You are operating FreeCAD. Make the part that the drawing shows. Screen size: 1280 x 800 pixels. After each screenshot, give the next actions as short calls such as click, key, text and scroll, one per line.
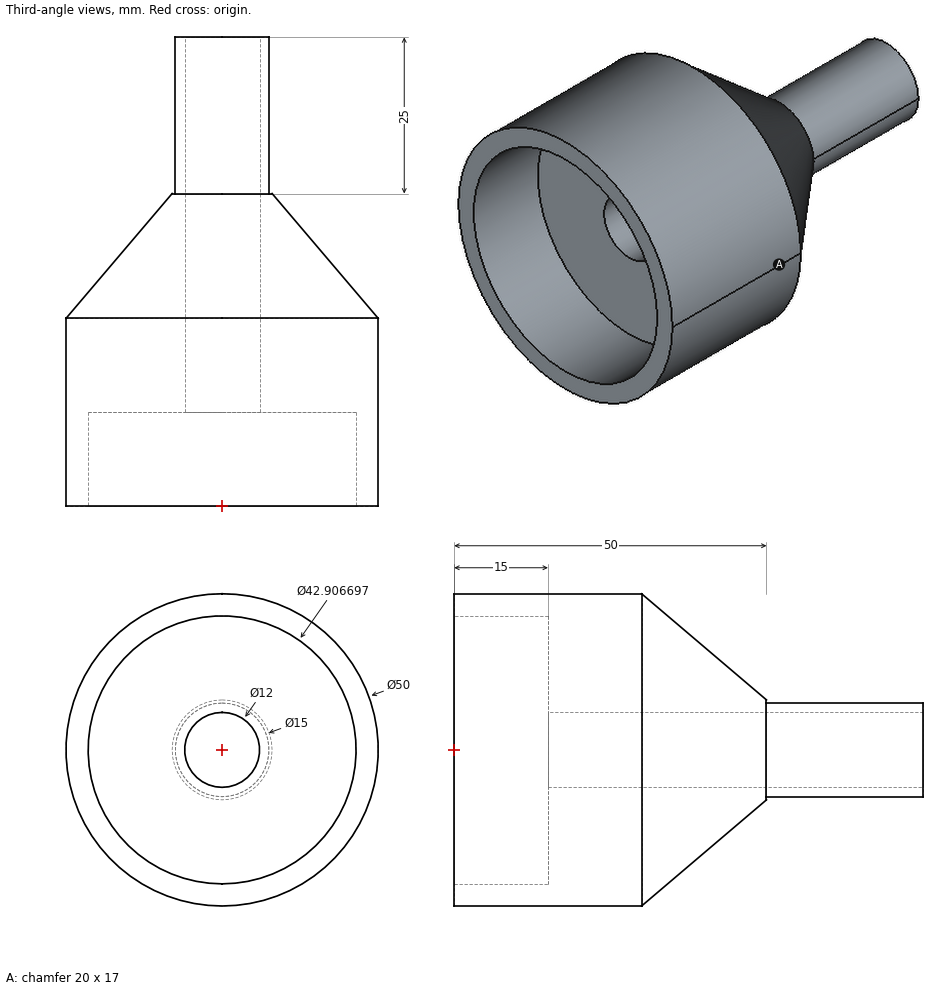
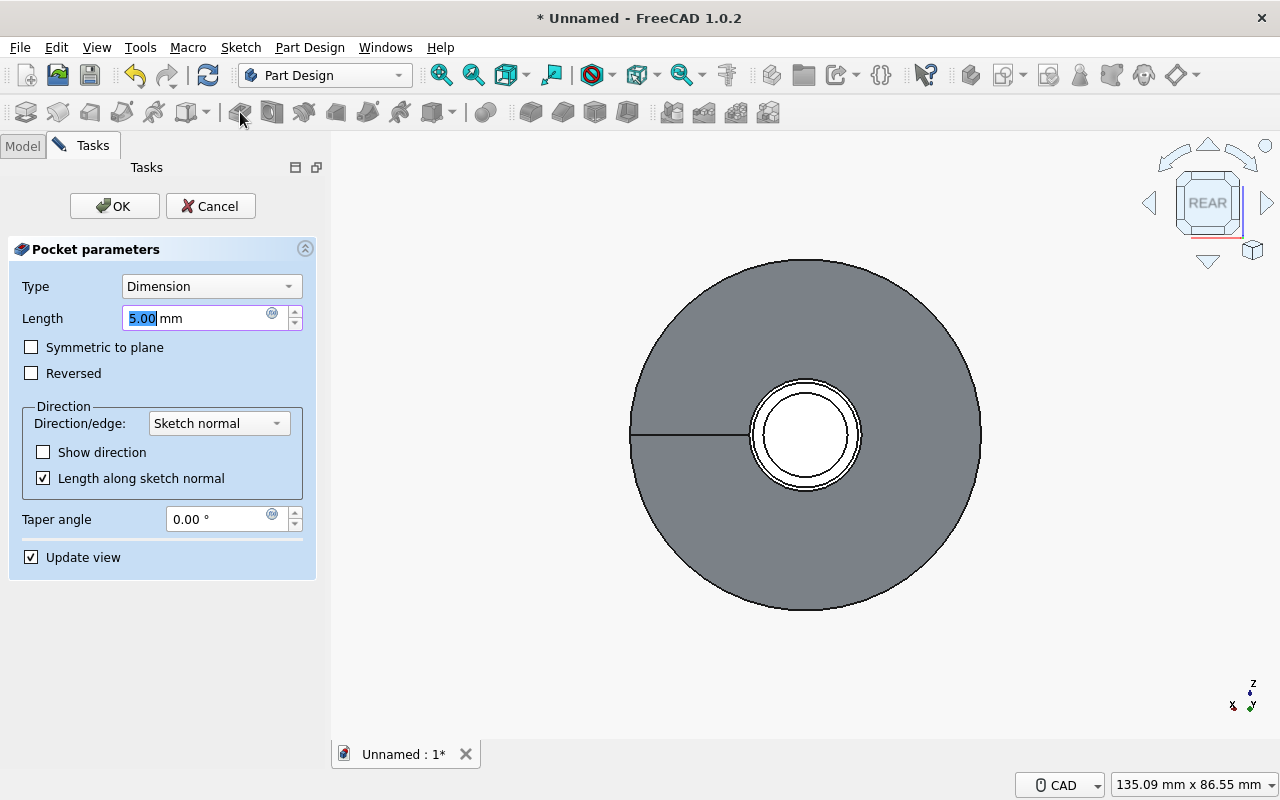
click(212, 286)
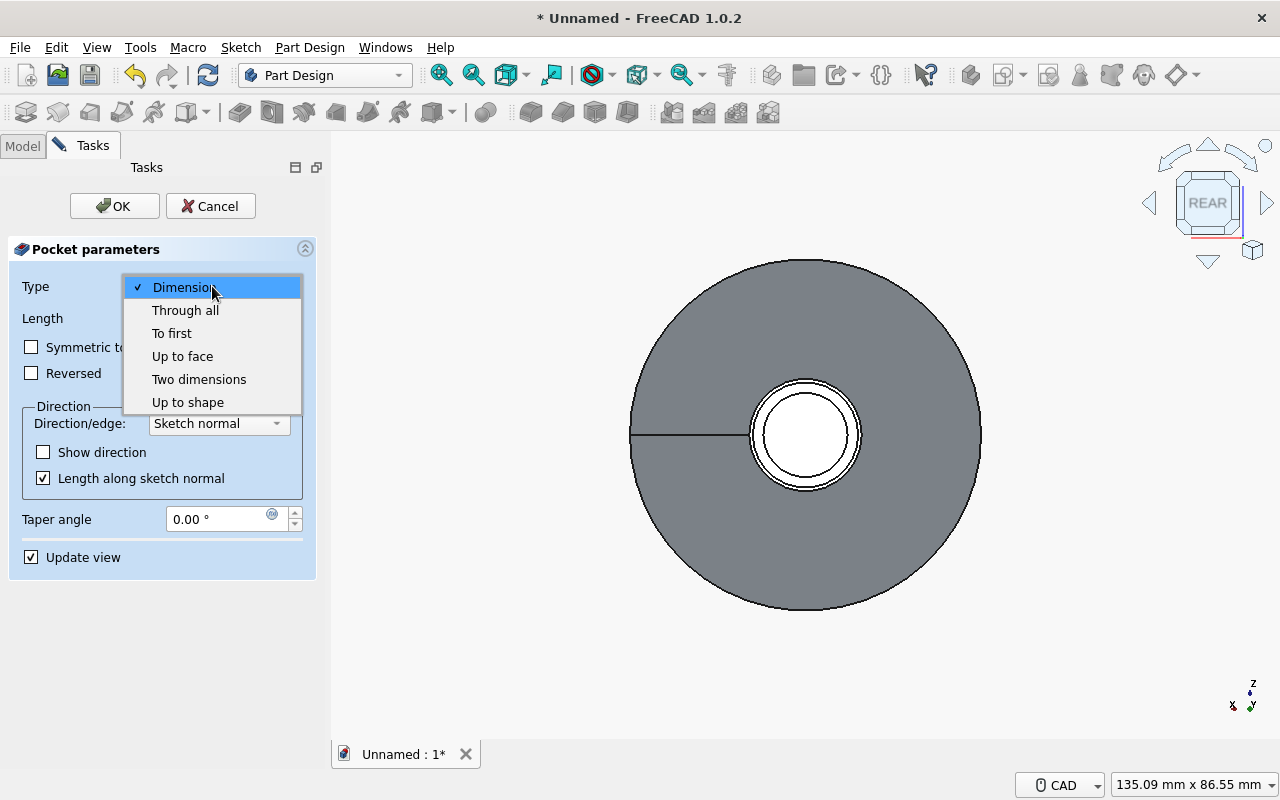
click(212, 310)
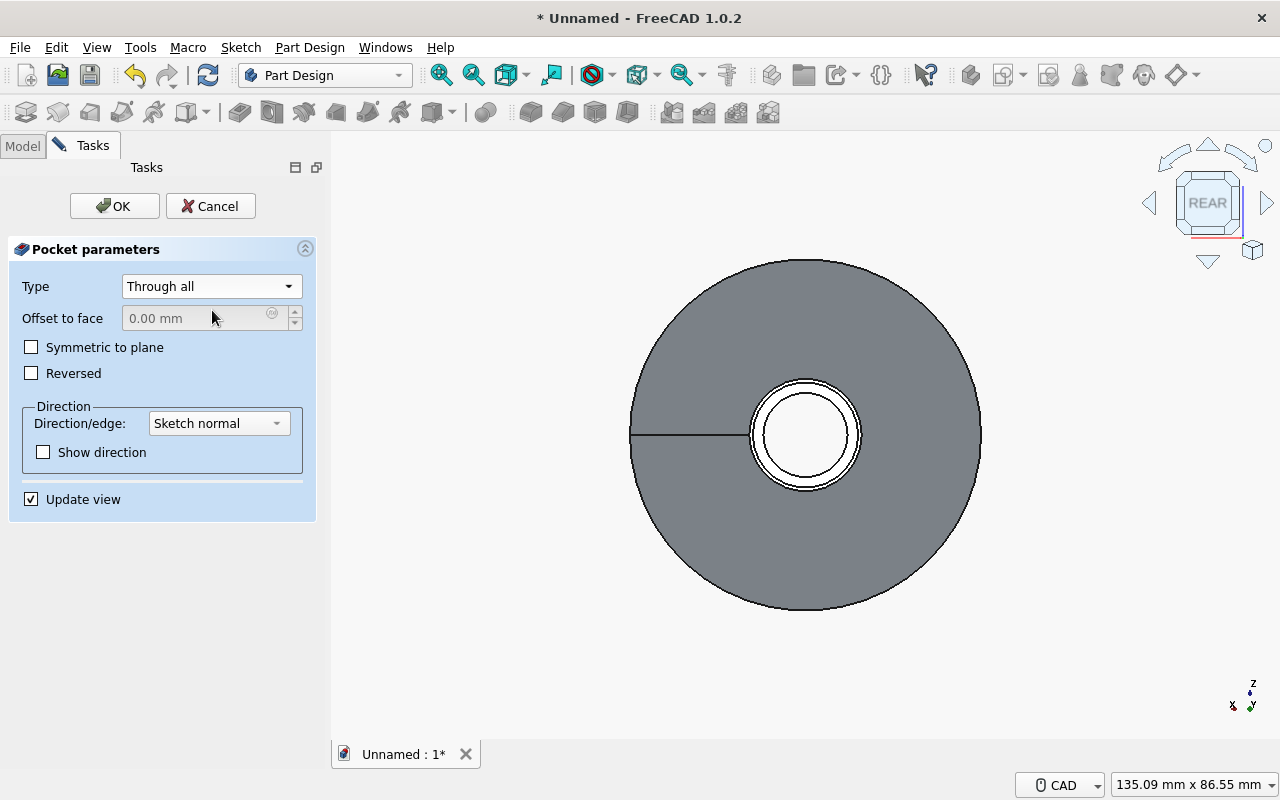
click(115, 206)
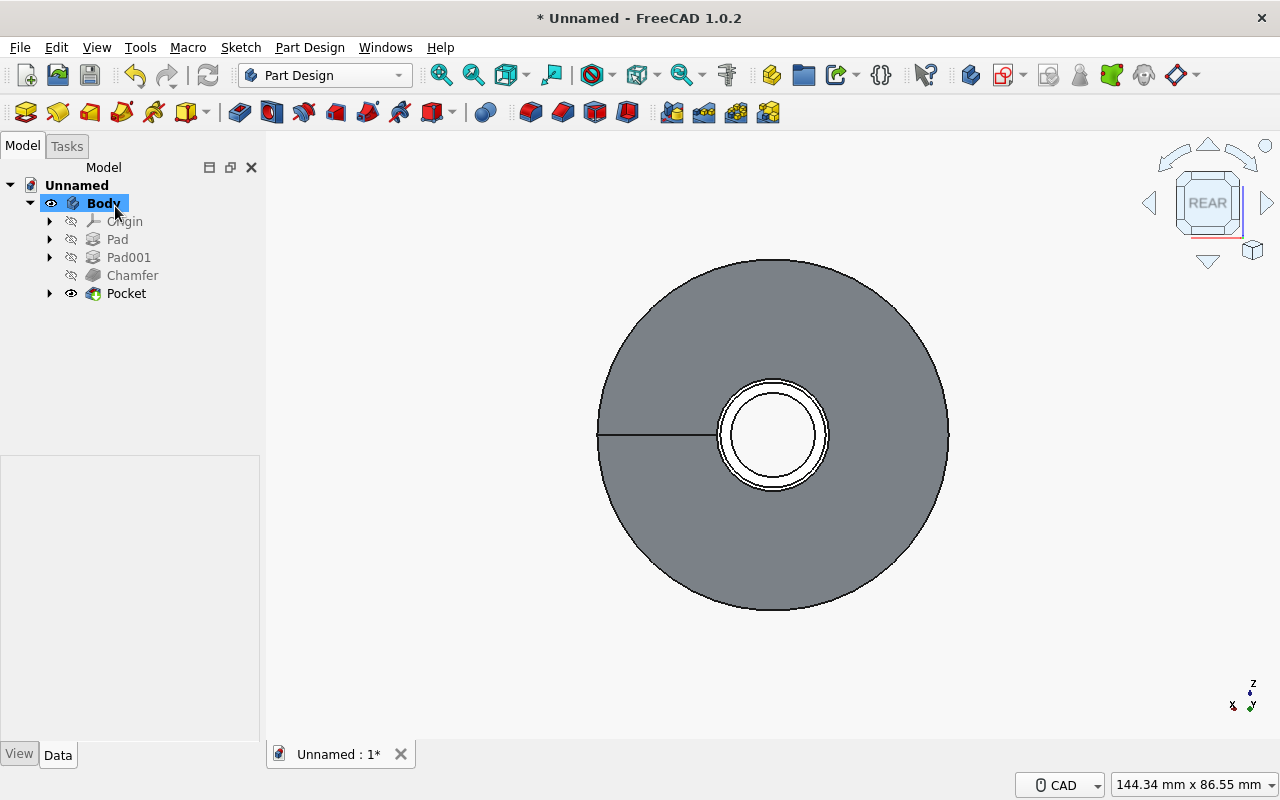
click(1004, 76)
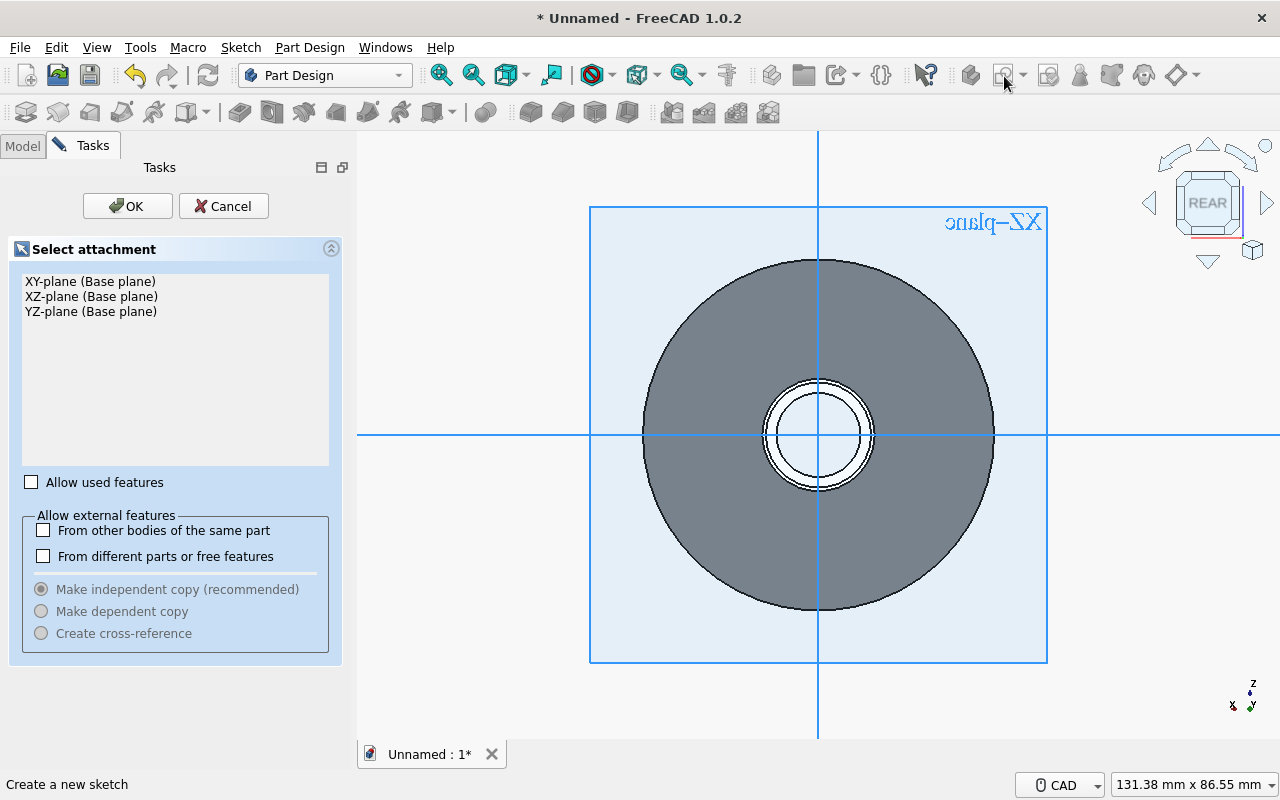
click(82, 296)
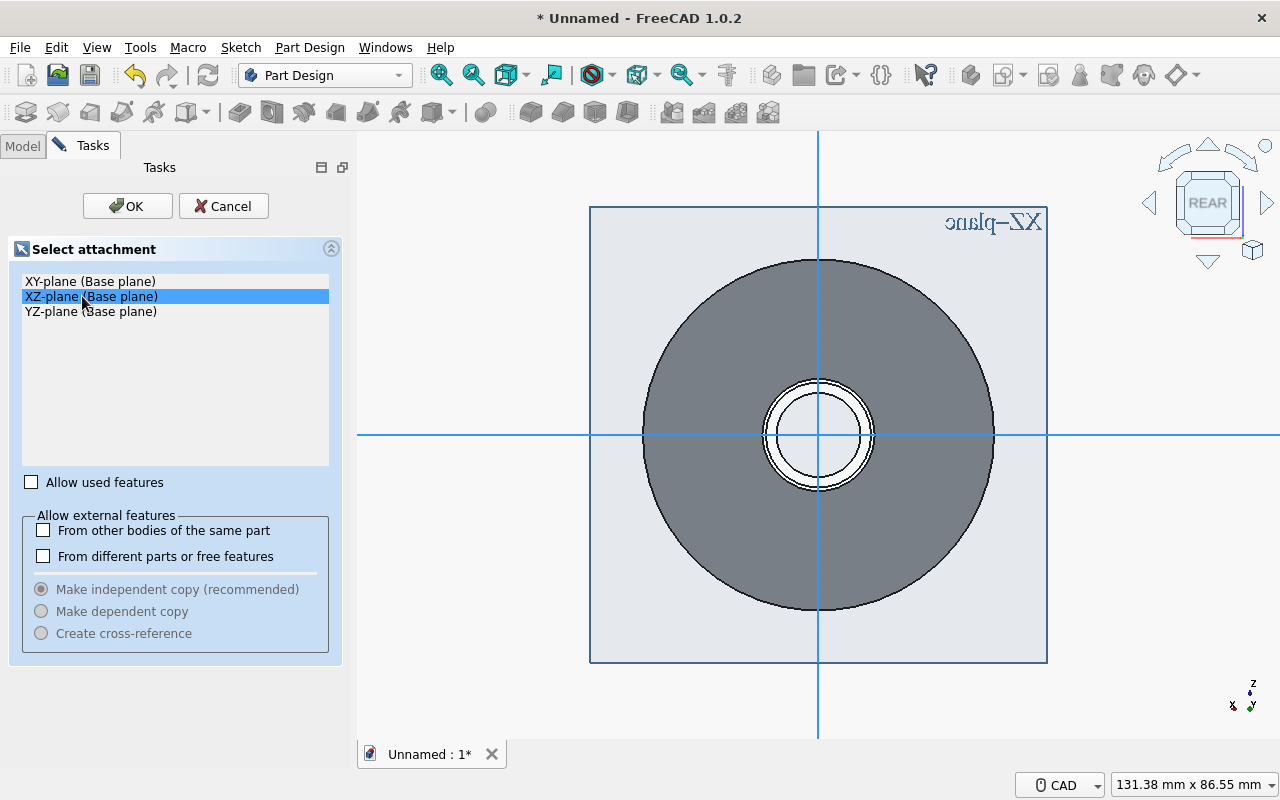
click(128, 206)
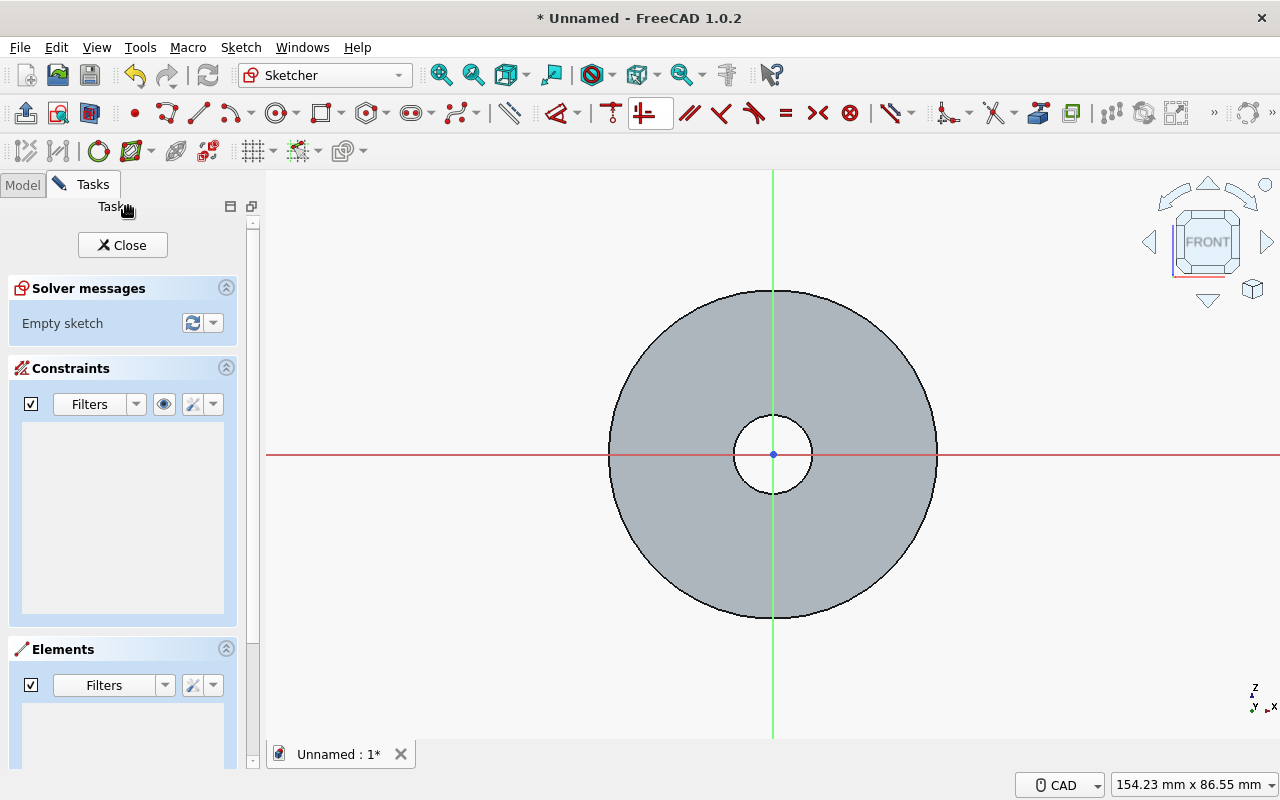
click(276, 114)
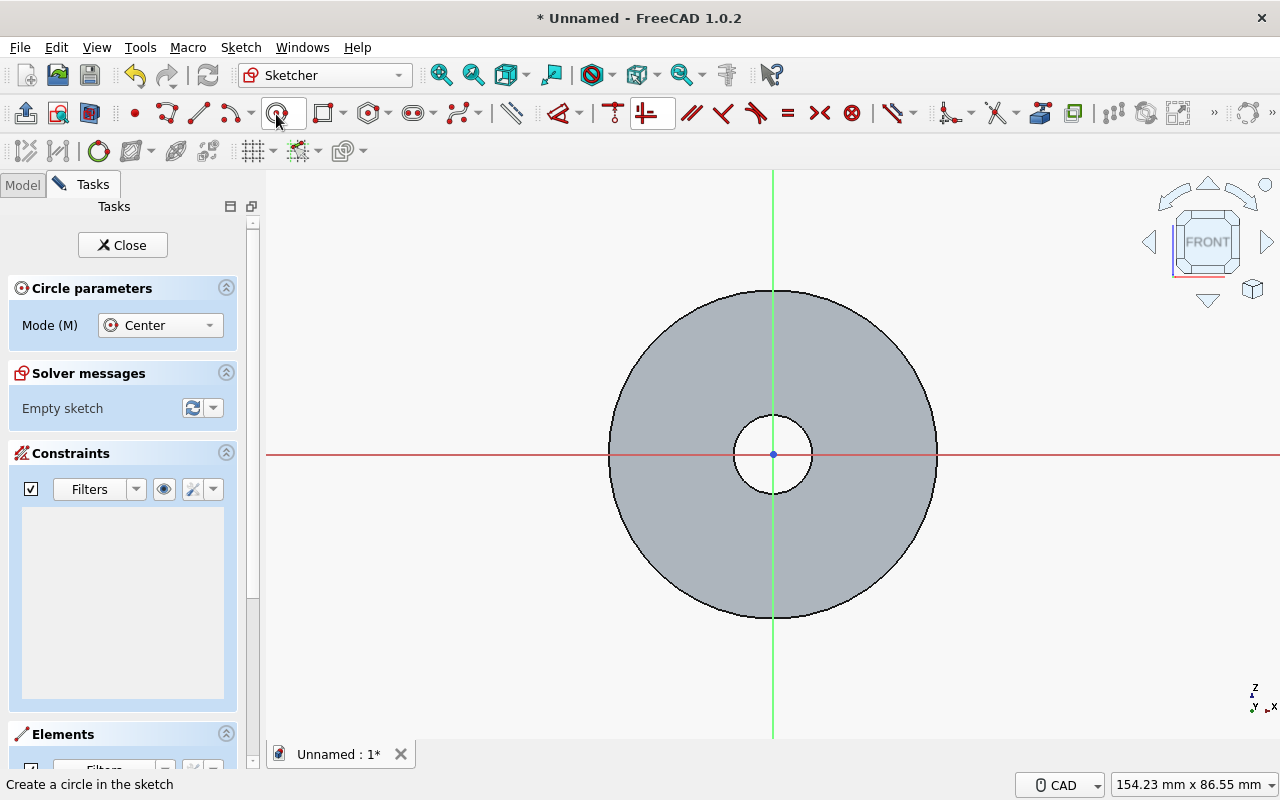
click(773, 455)
move(873, 355)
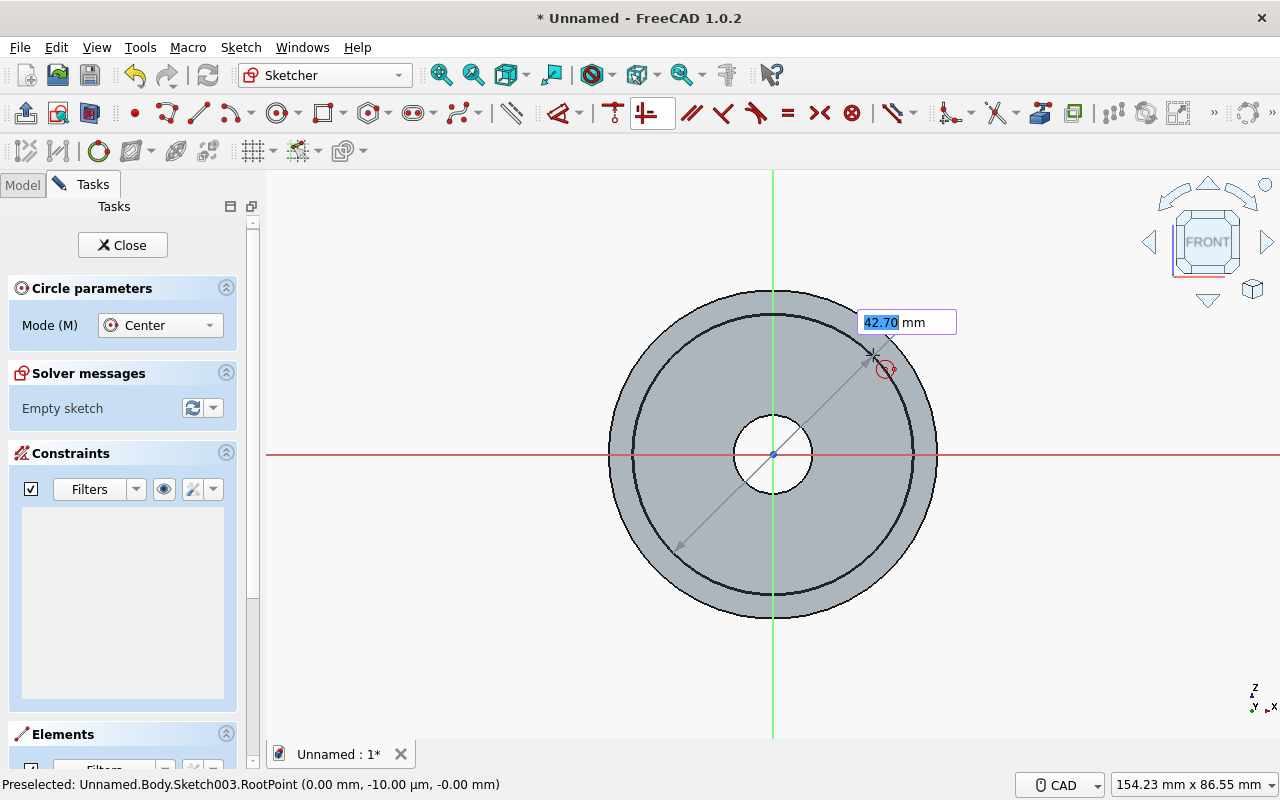
text(42.906697)
key(Return)
key(Escape)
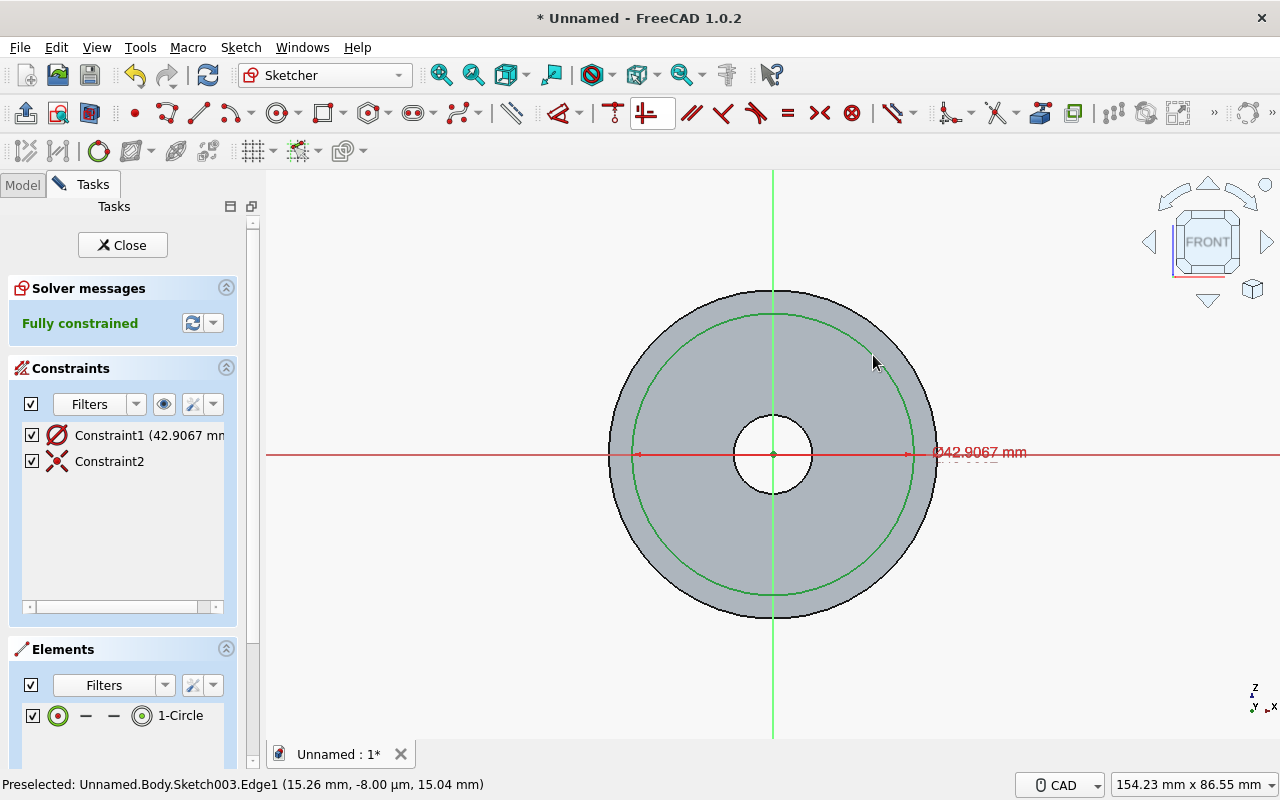
click(123, 245)